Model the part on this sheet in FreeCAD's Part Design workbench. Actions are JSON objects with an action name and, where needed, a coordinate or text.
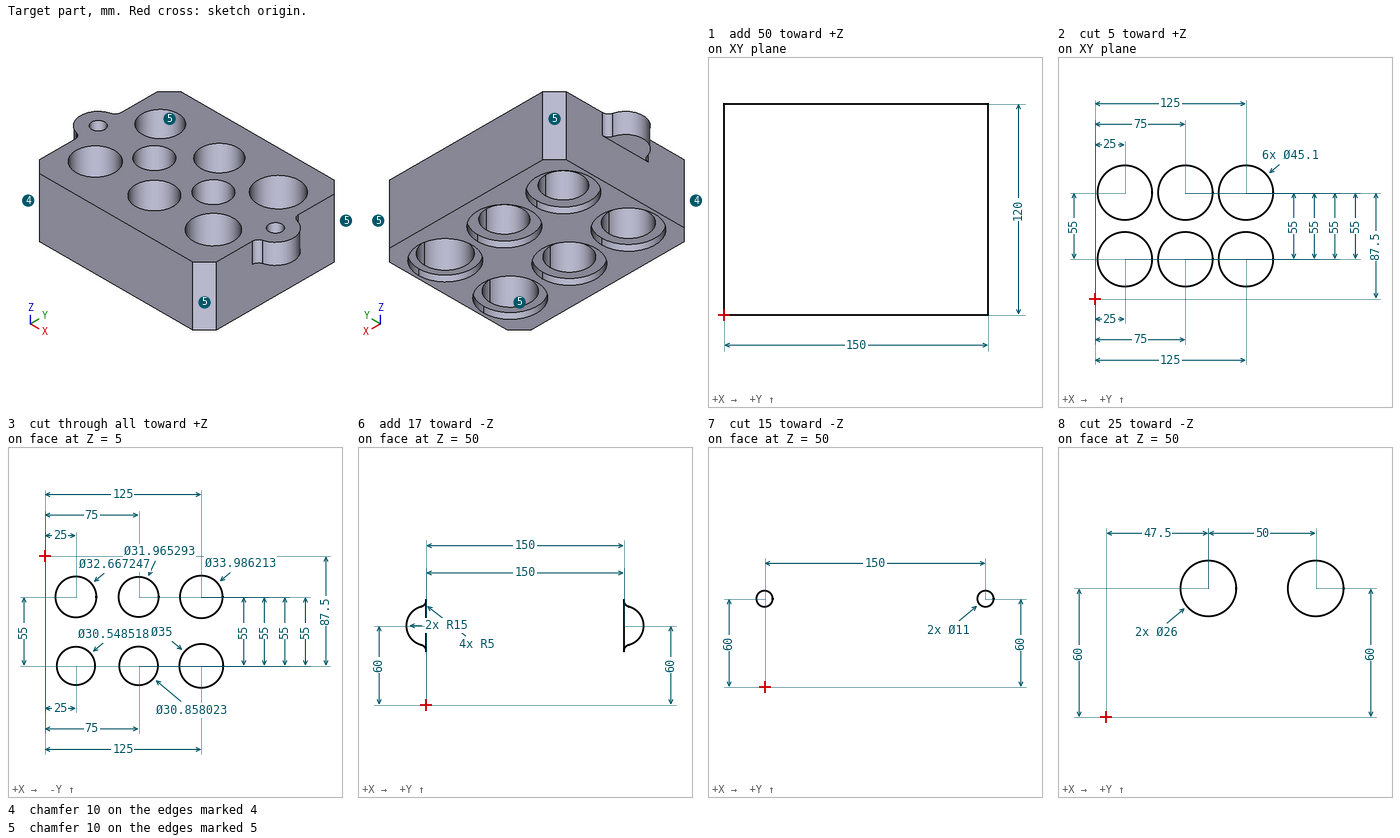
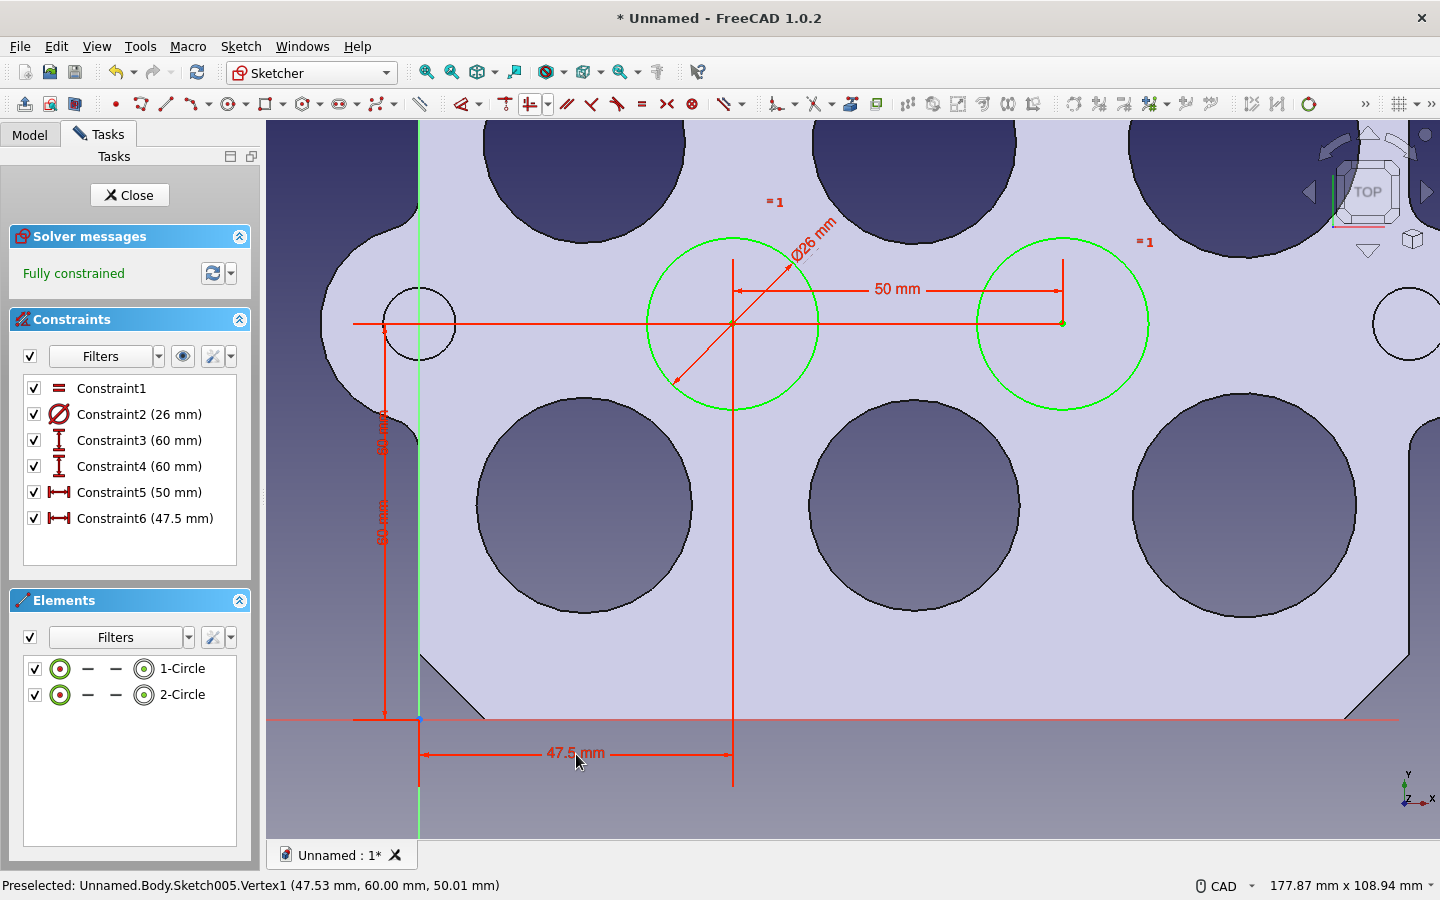
{"action": "left_click", "coordinate": [130, 195]}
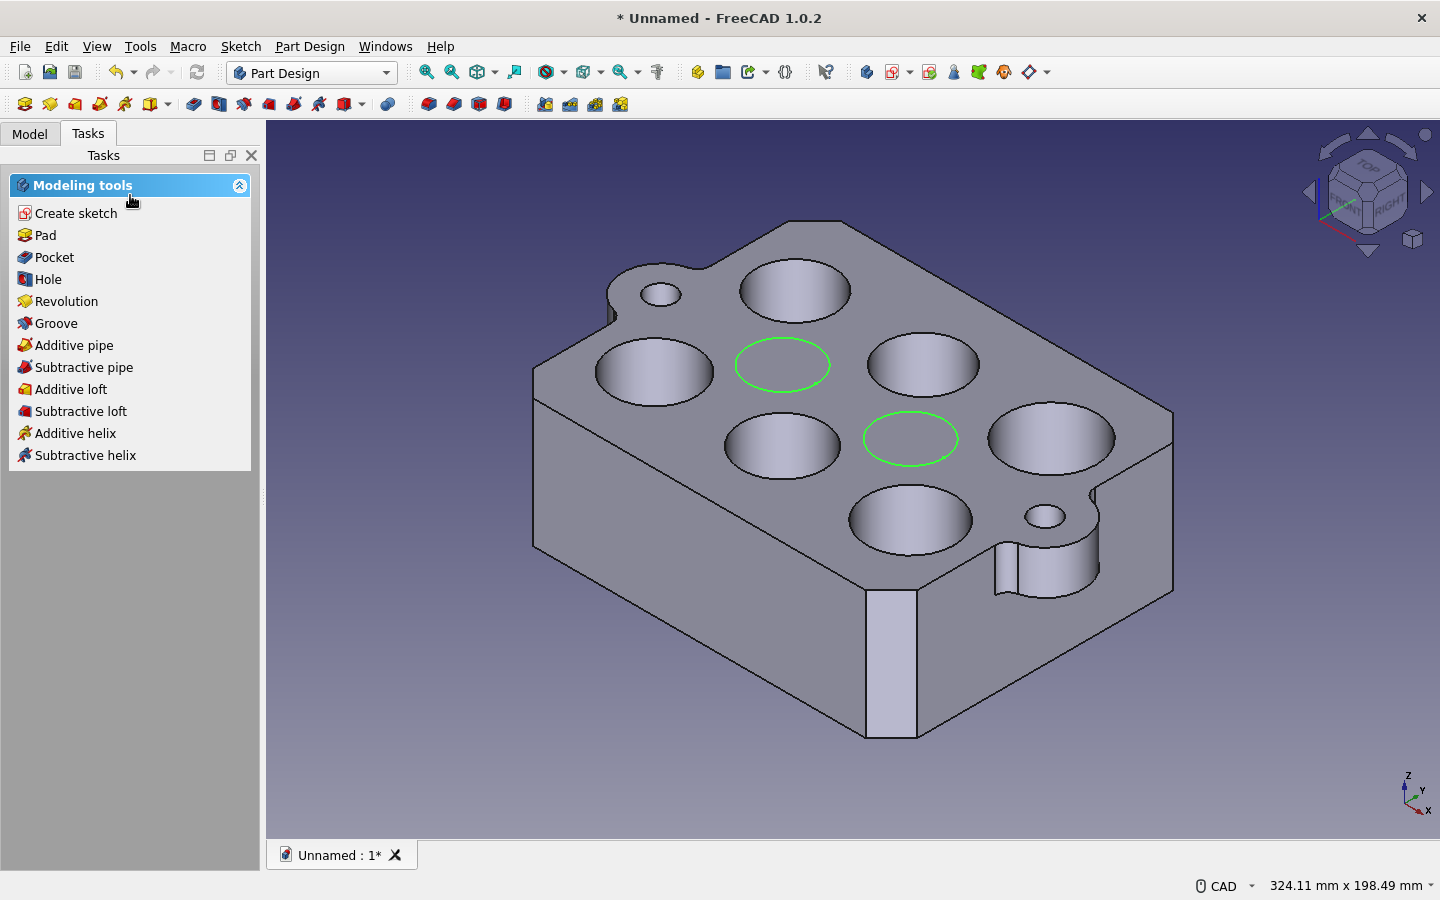
{"action": "left_click", "coordinate": [194, 104]}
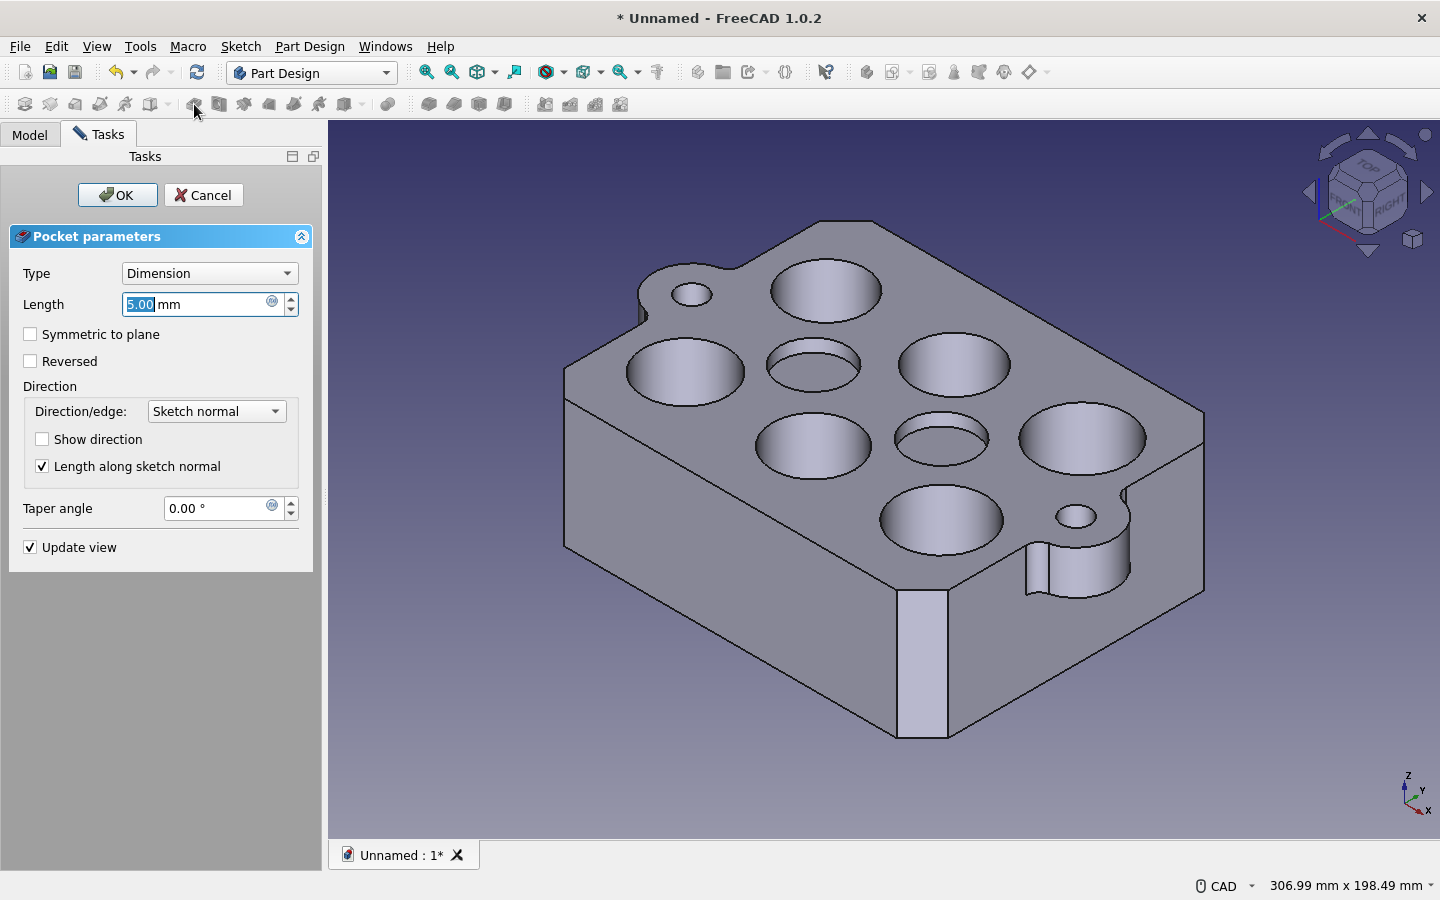
{"action": "type", "text": "25"}
{"action": "key", "text": "Tab"}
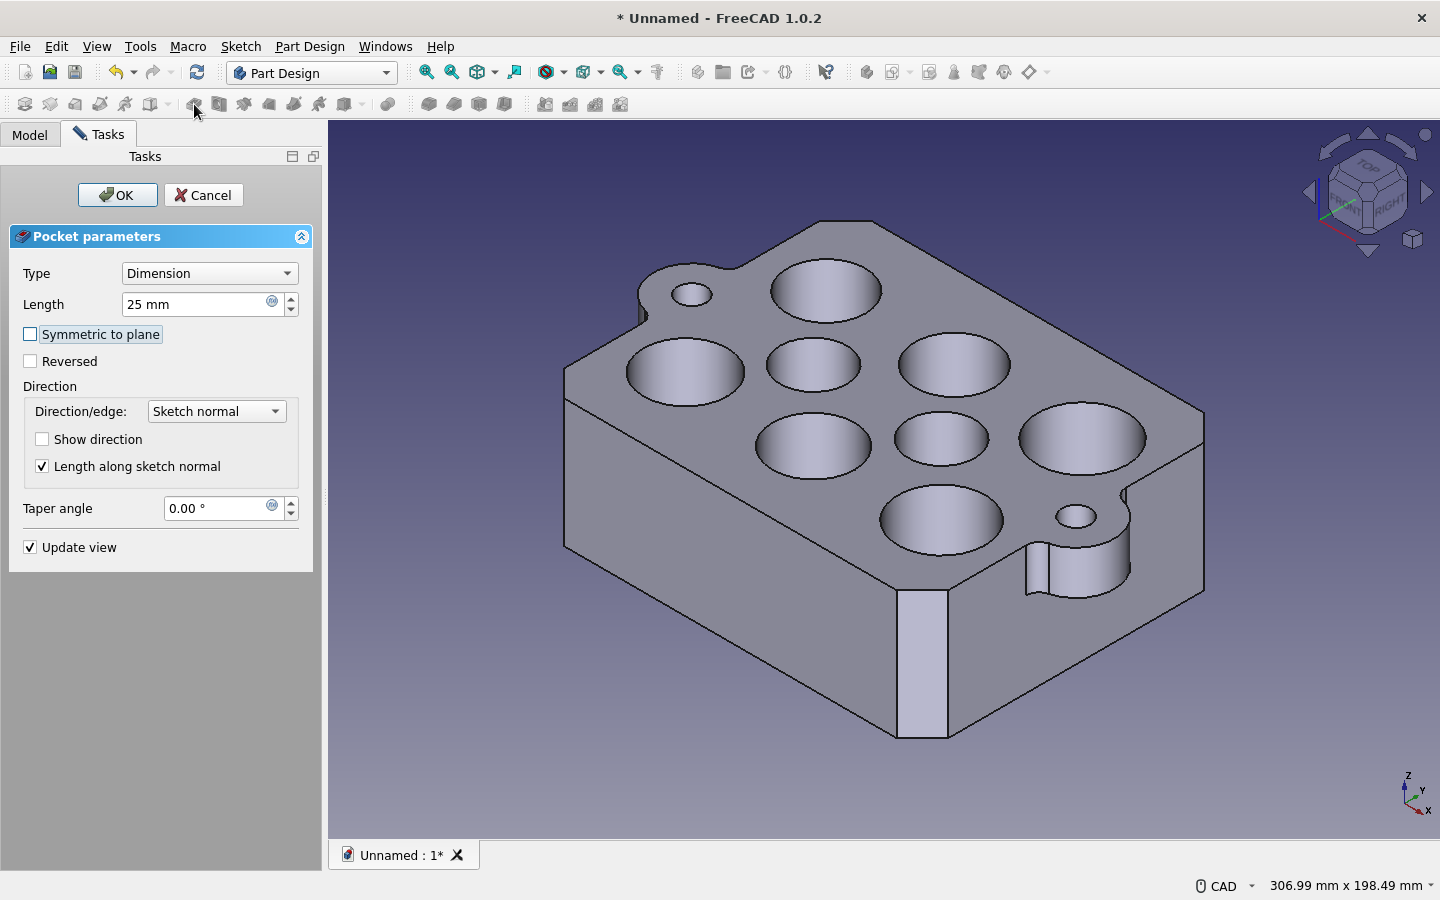
{"action": "left_click", "coordinate": [118, 195]}